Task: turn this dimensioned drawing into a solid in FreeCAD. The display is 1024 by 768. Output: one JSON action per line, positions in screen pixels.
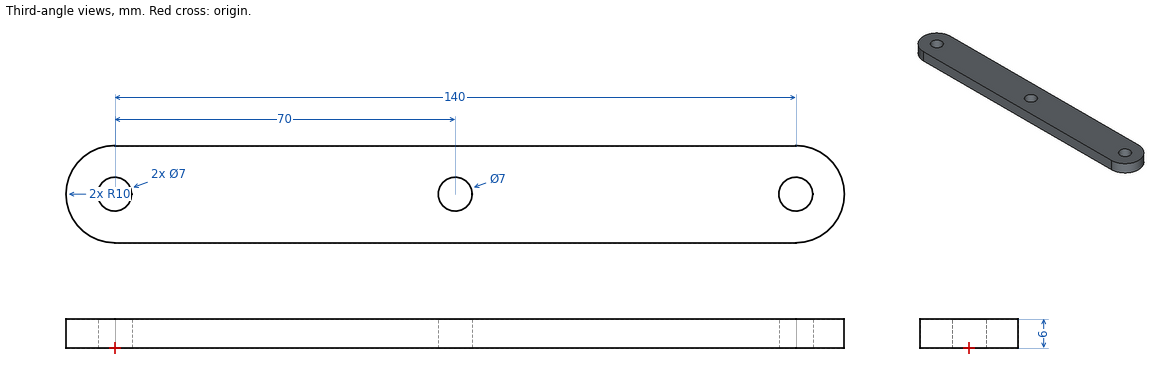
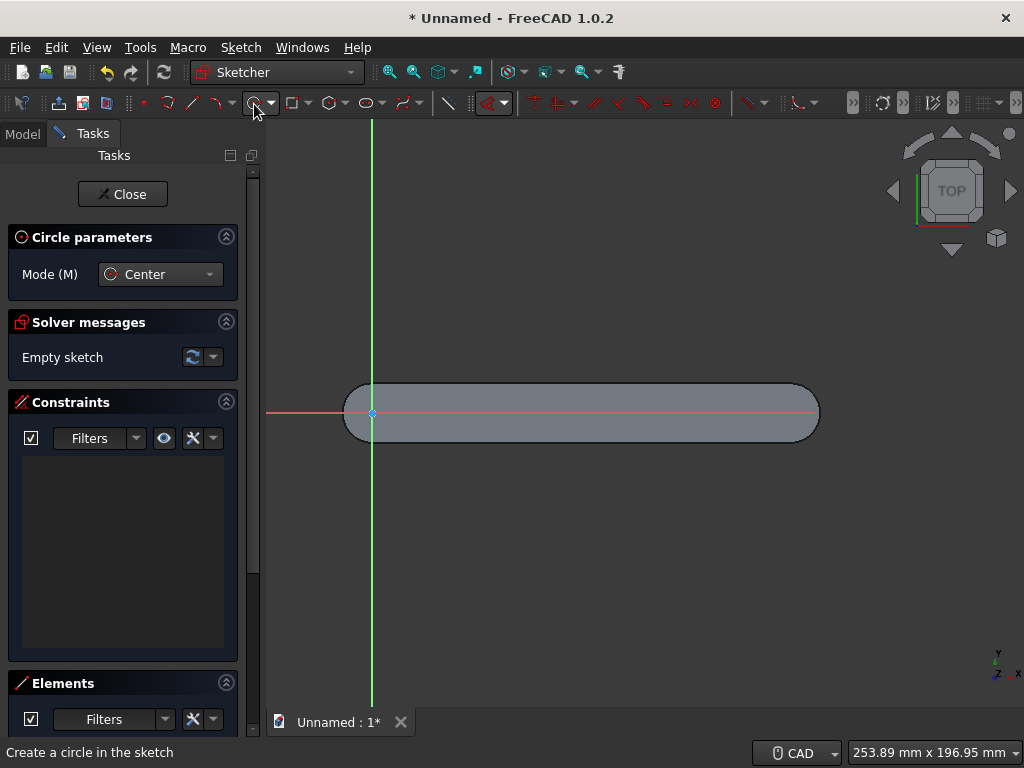
{"action": "scroll", "coordinate": [372, 413], "scroll_direction": "up", "scroll_amount": 4}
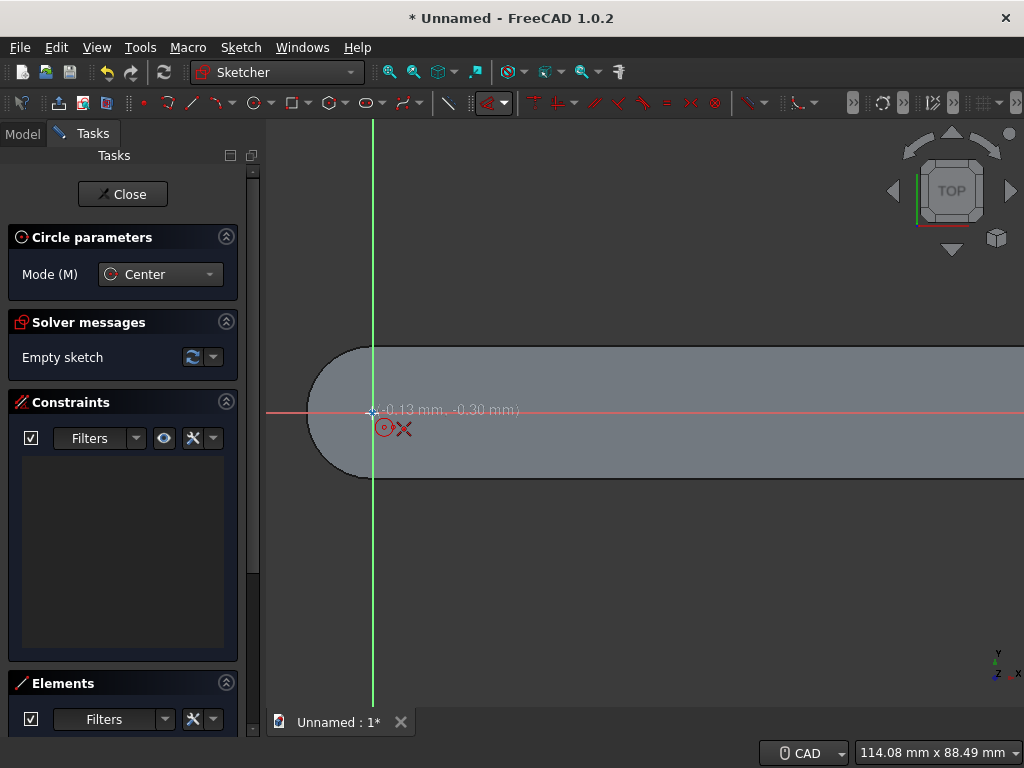
{"action": "left_click", "coordinate": [373, 413]}
{"action": "mouse_move", "coordinate": [389, 396]}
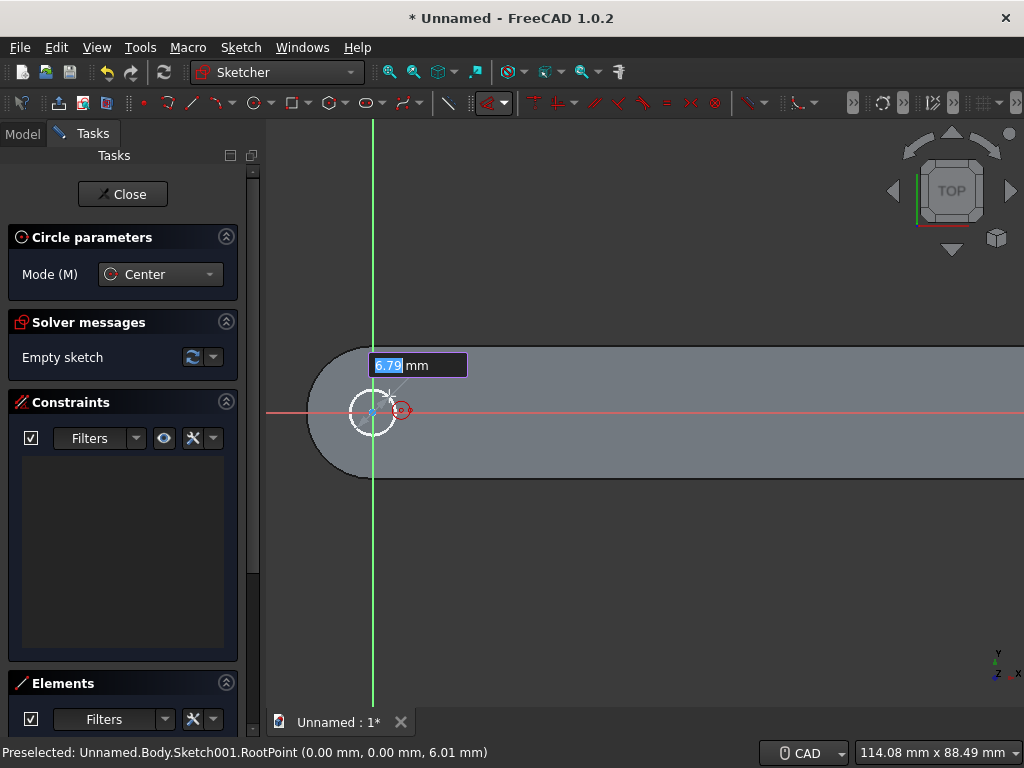
{"action": "type", "text": "7"}
{"action": "key", "text": "Return"}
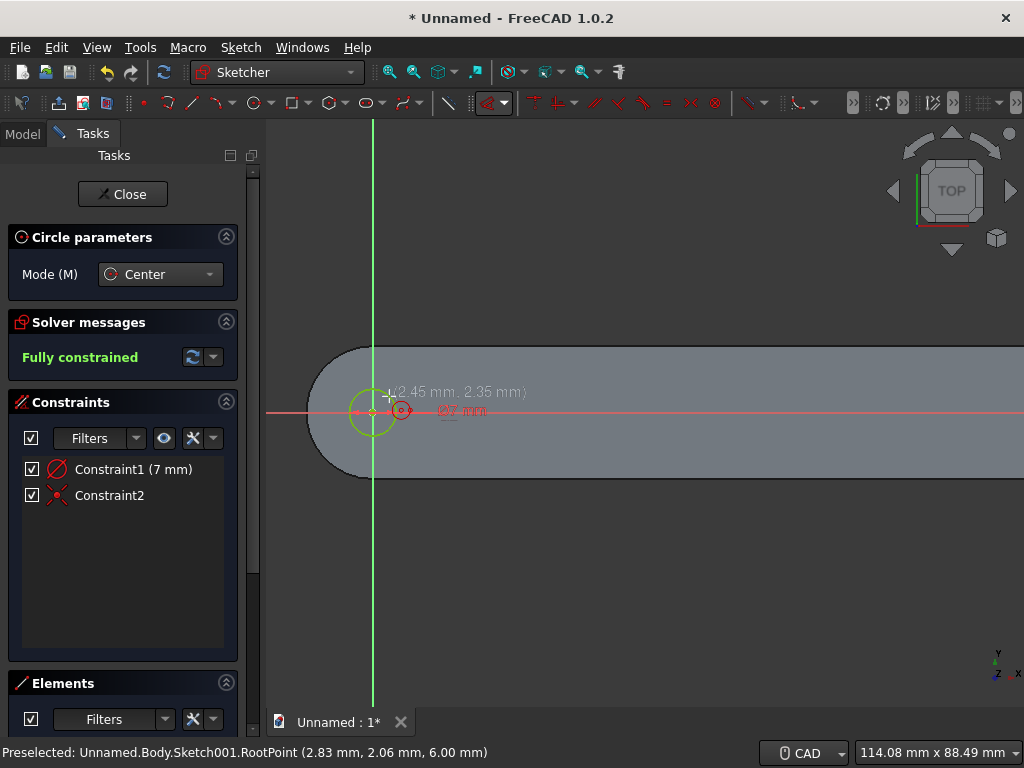
{"action": "scroll", "coordinate": [363, 413], "scroll_direction": "down", "scroll_amount": 4}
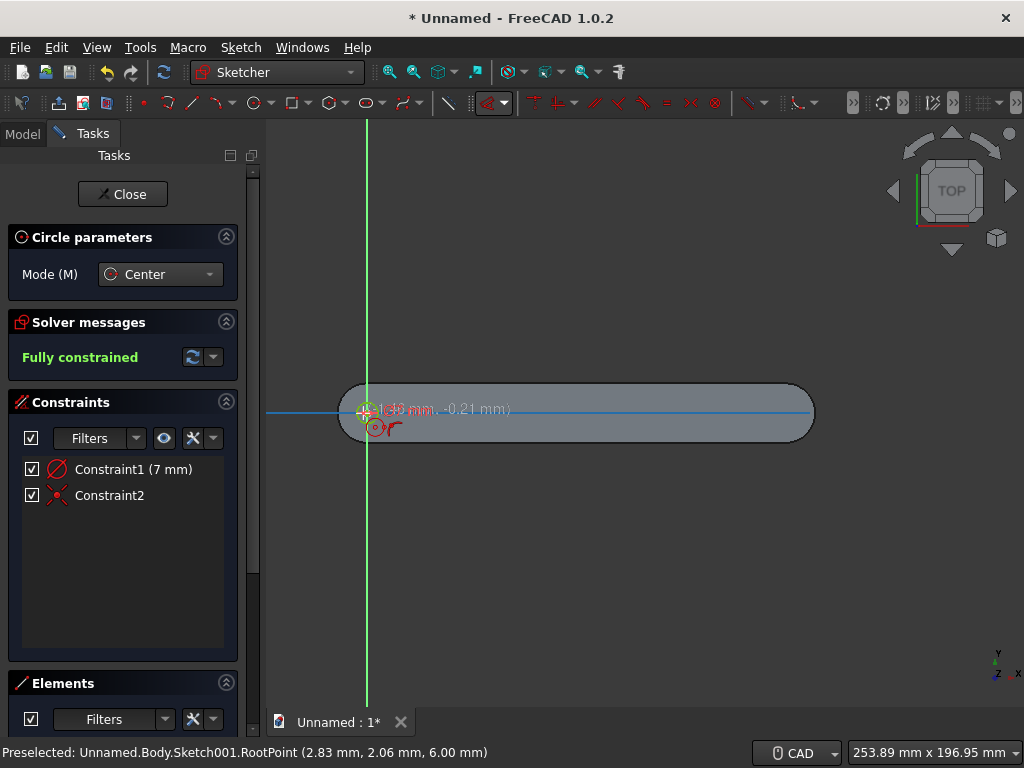
{"action": "scroll", "coordinate": [785, 413], "scroll_direction": "up", "scroll_amount": 4}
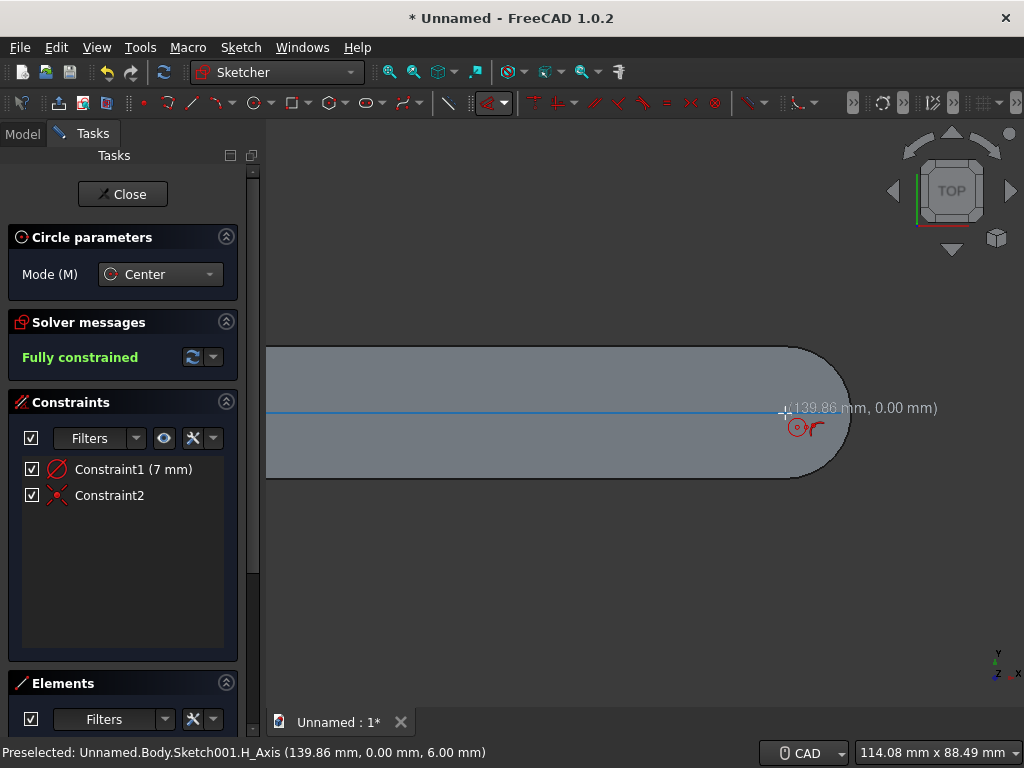
{"action": "left_click", "coordinate": [785, 413]}
{"action": "mouse_move", "coordinate": [802, 396]}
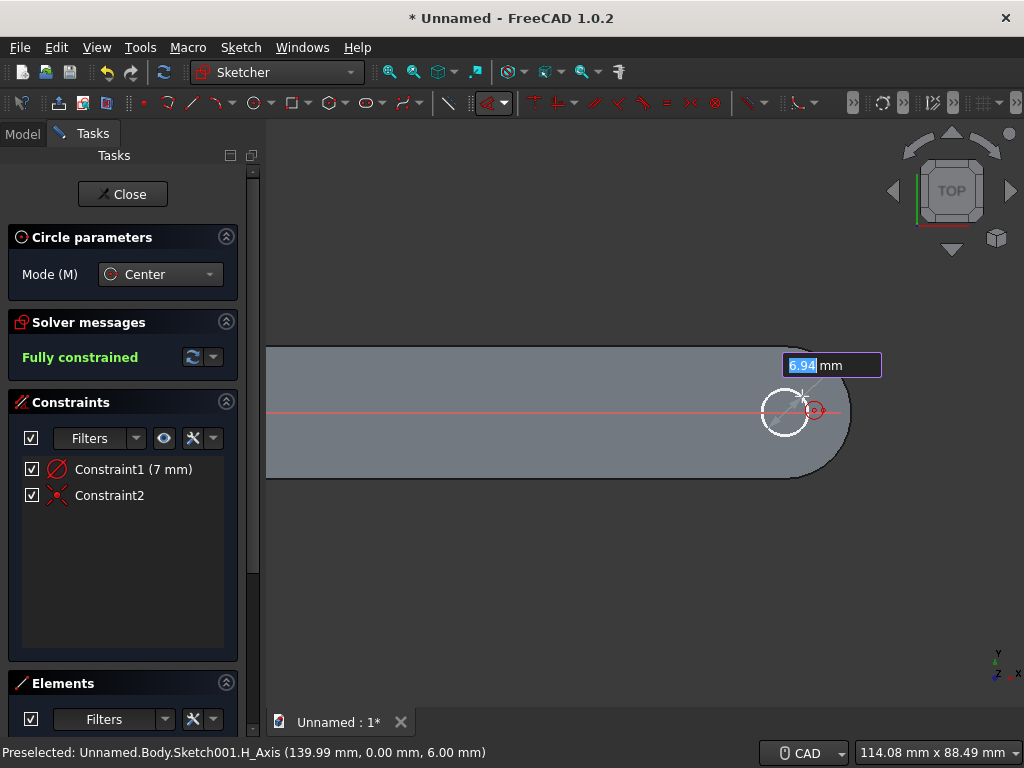
{"action": "type", "text": "7"}
{"action": "key", "text": "Return"}
{"action": "key", "text": "Escape"}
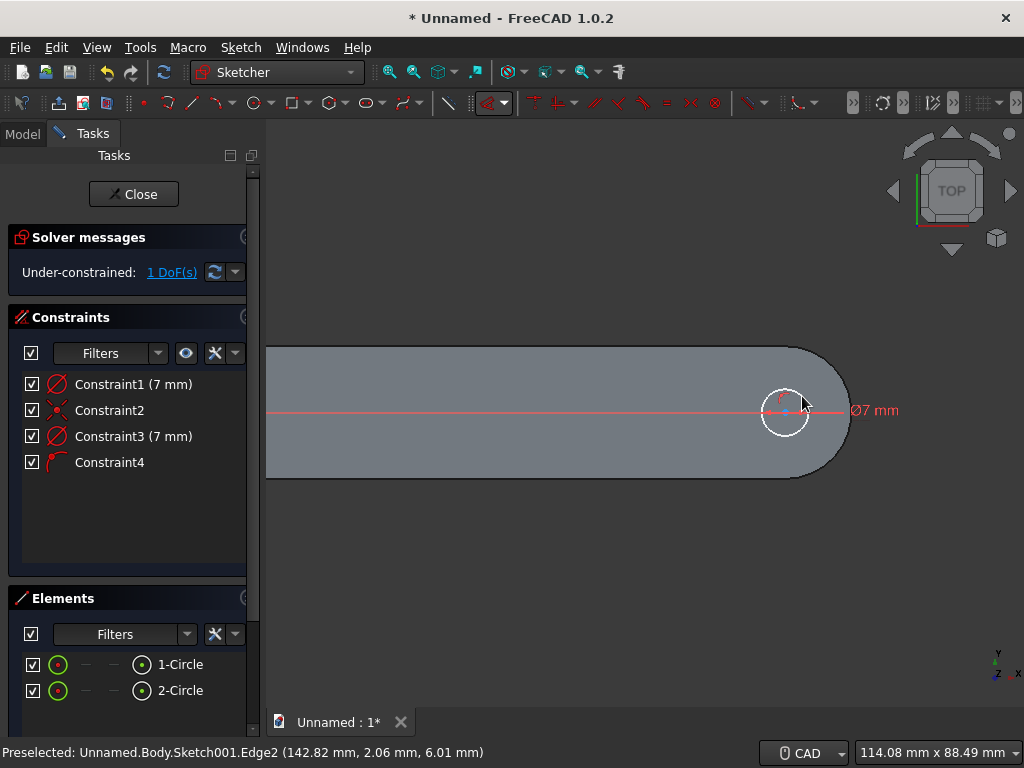
{"action": "left_click", "coordinate": [785, 413]}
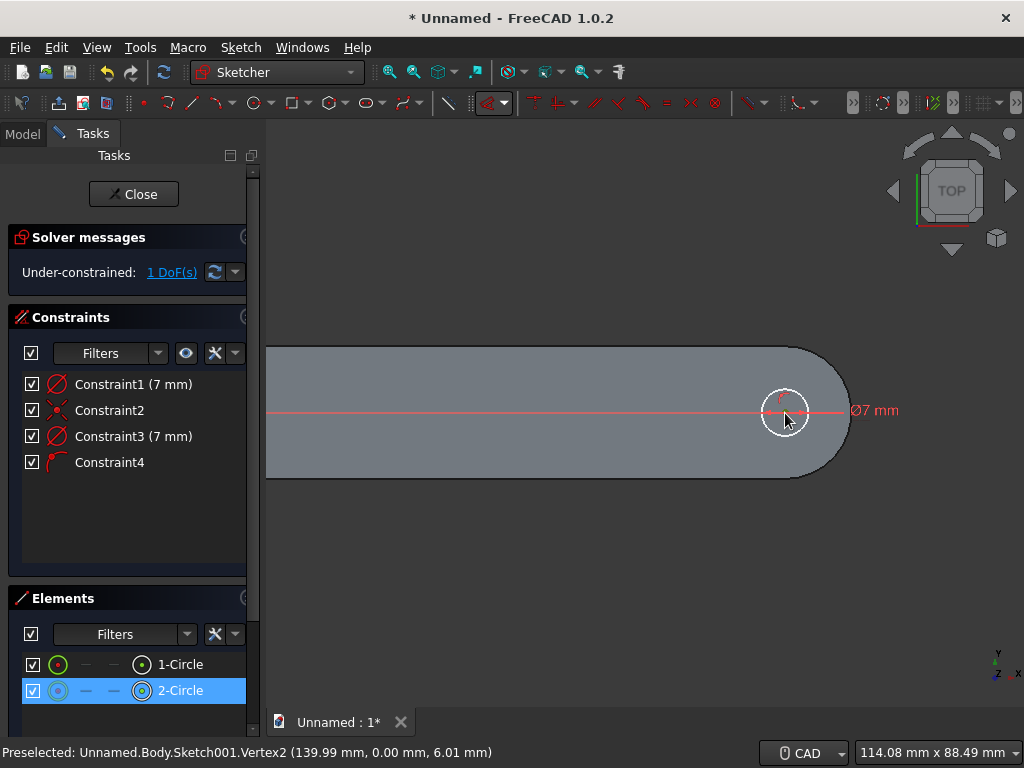
{"action": "key", "text": "l"}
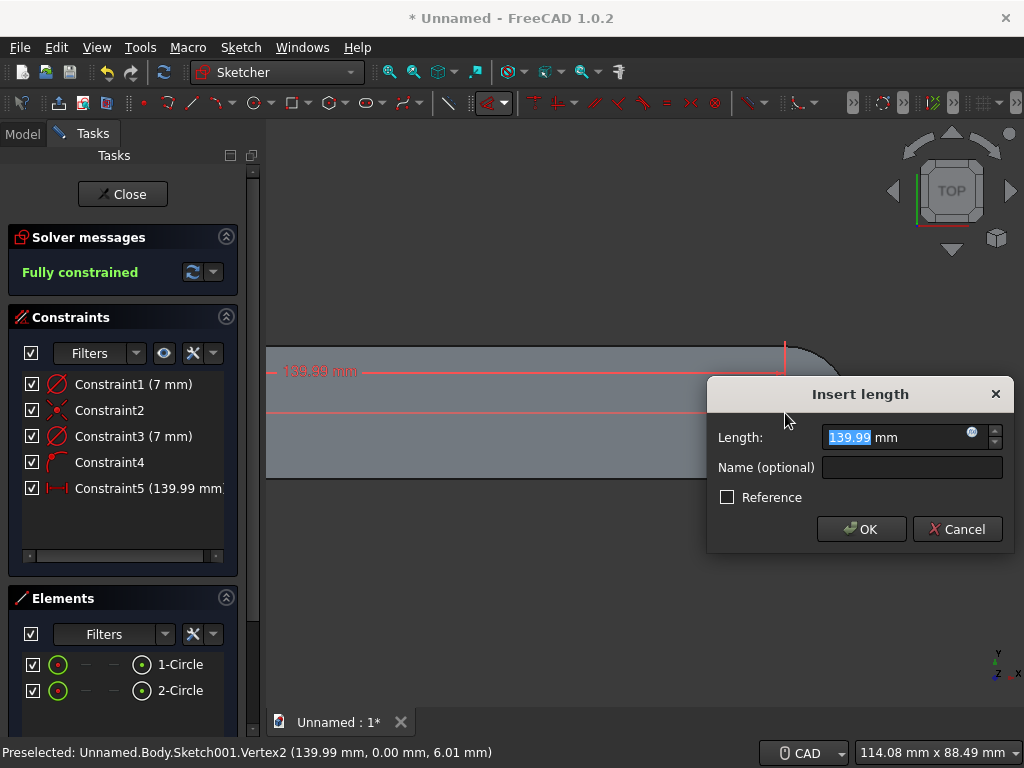
{"action": "type", "text": "140"}
{"action": "key", "text": "Return"}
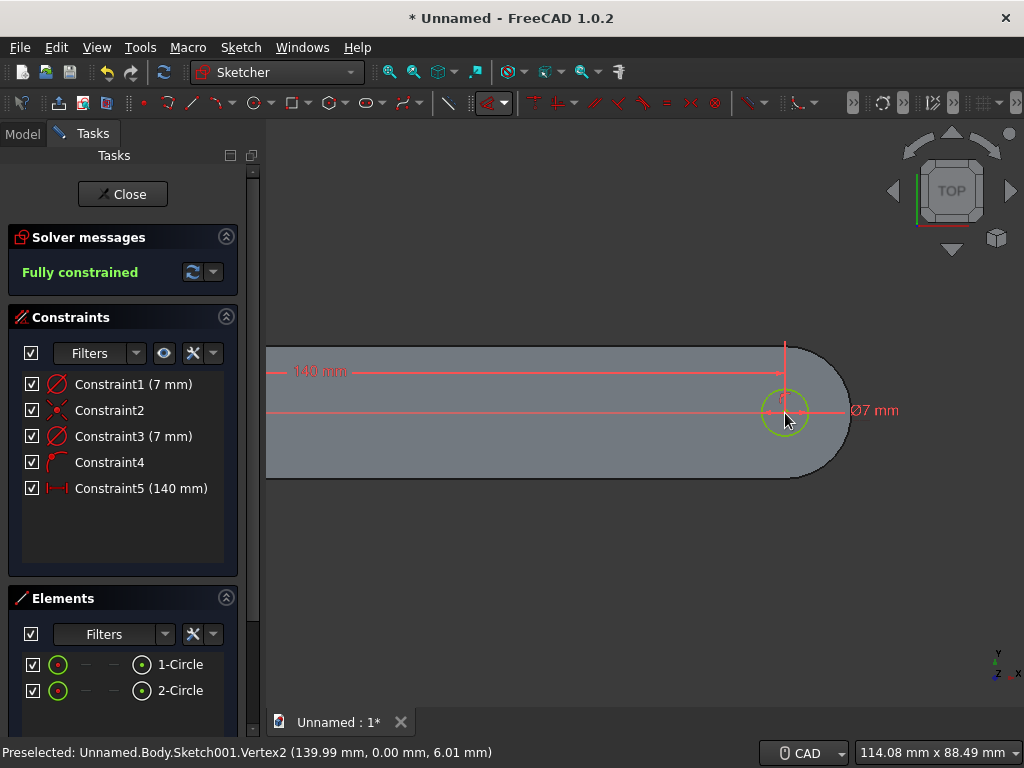
{"action": "left_click", "coordinate": [123, 194]}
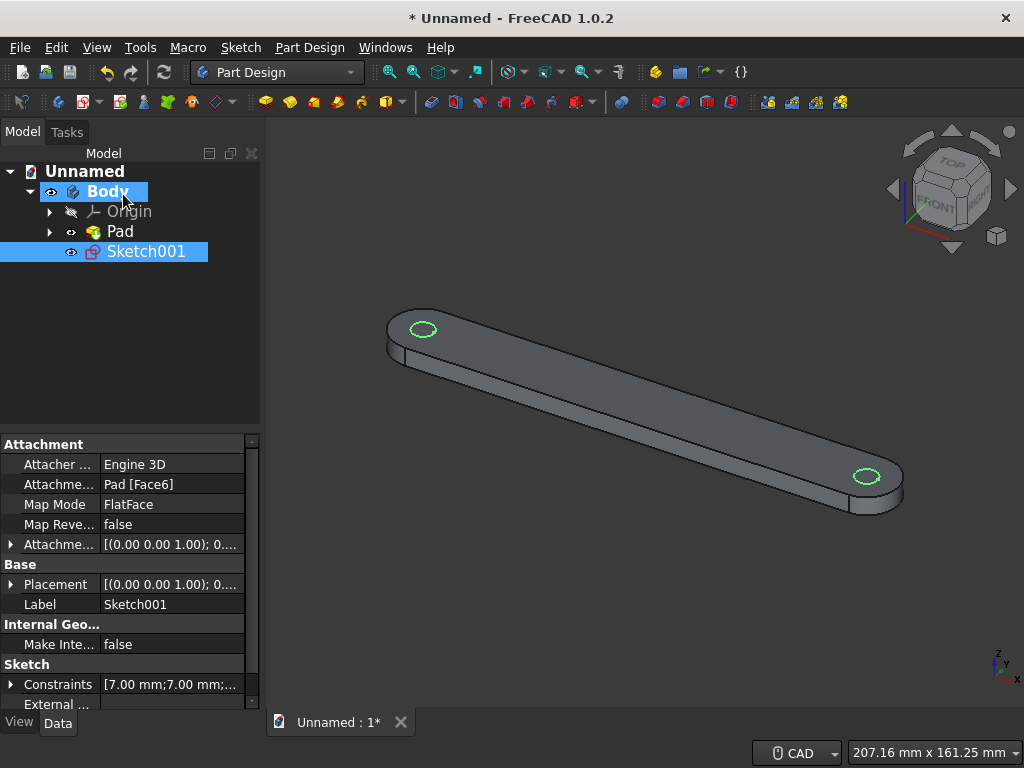
{"action": "left_click", "coordinate": [432, 102]}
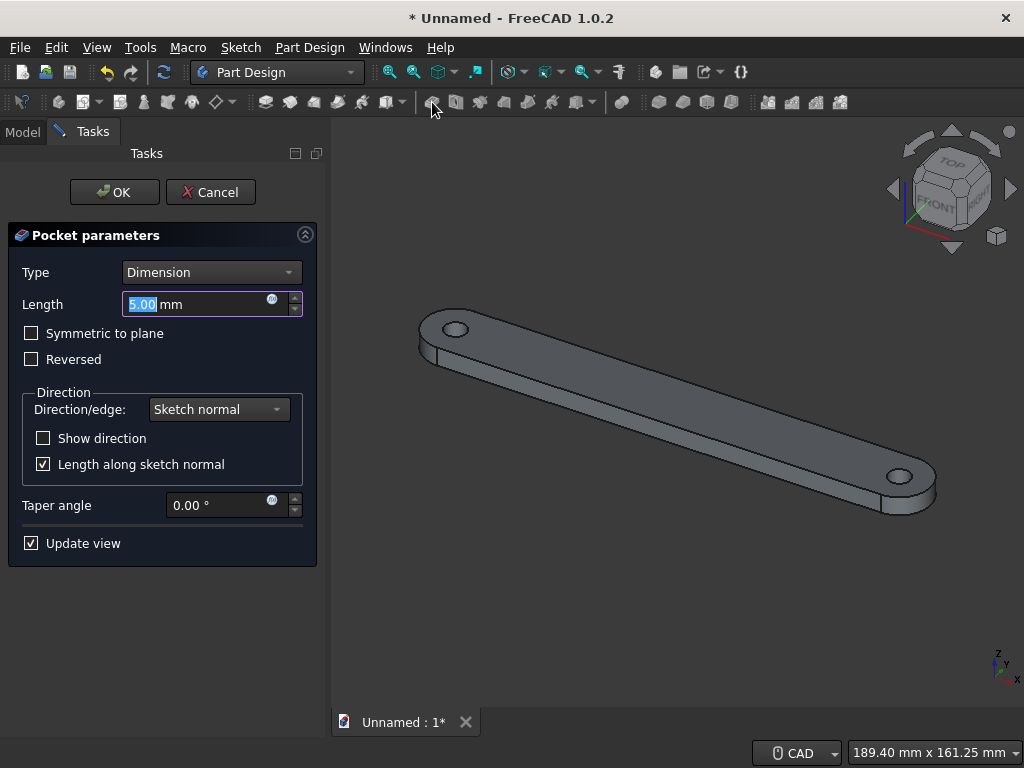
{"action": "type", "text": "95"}
{"action": "key", "text": "Tab"}